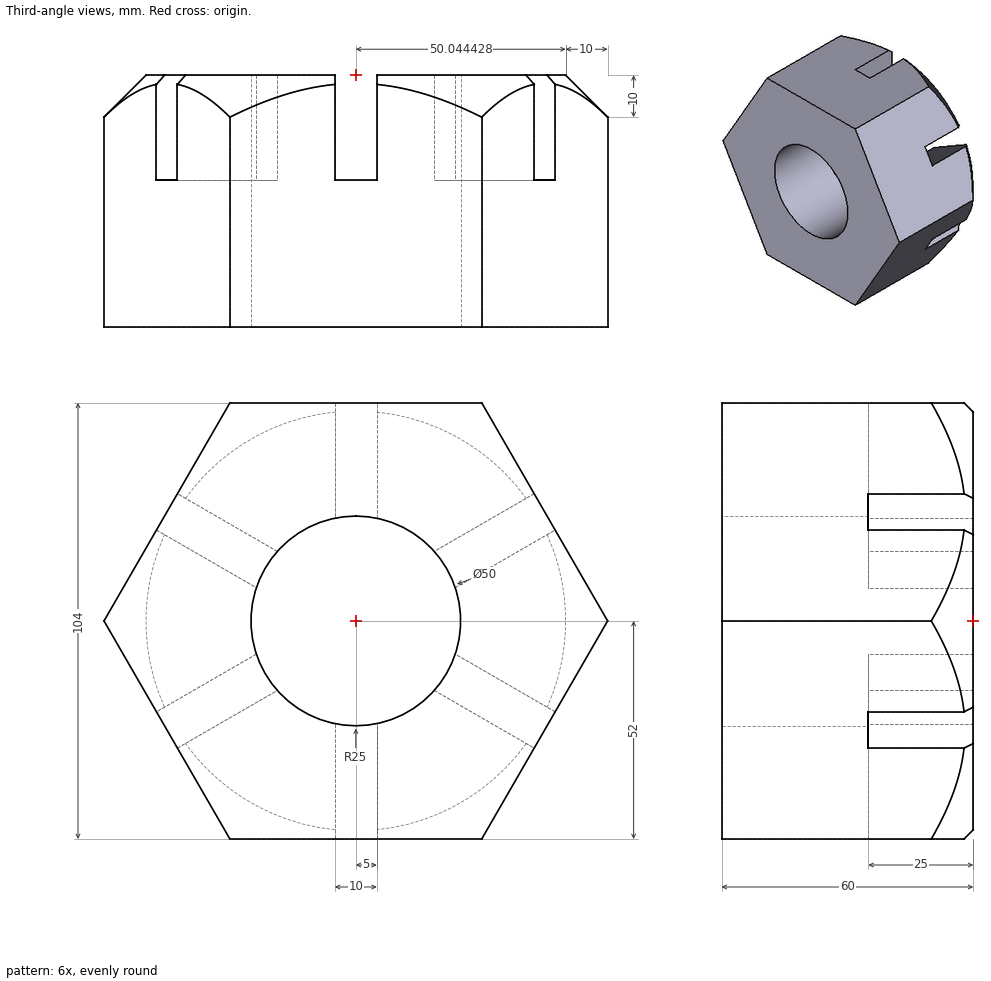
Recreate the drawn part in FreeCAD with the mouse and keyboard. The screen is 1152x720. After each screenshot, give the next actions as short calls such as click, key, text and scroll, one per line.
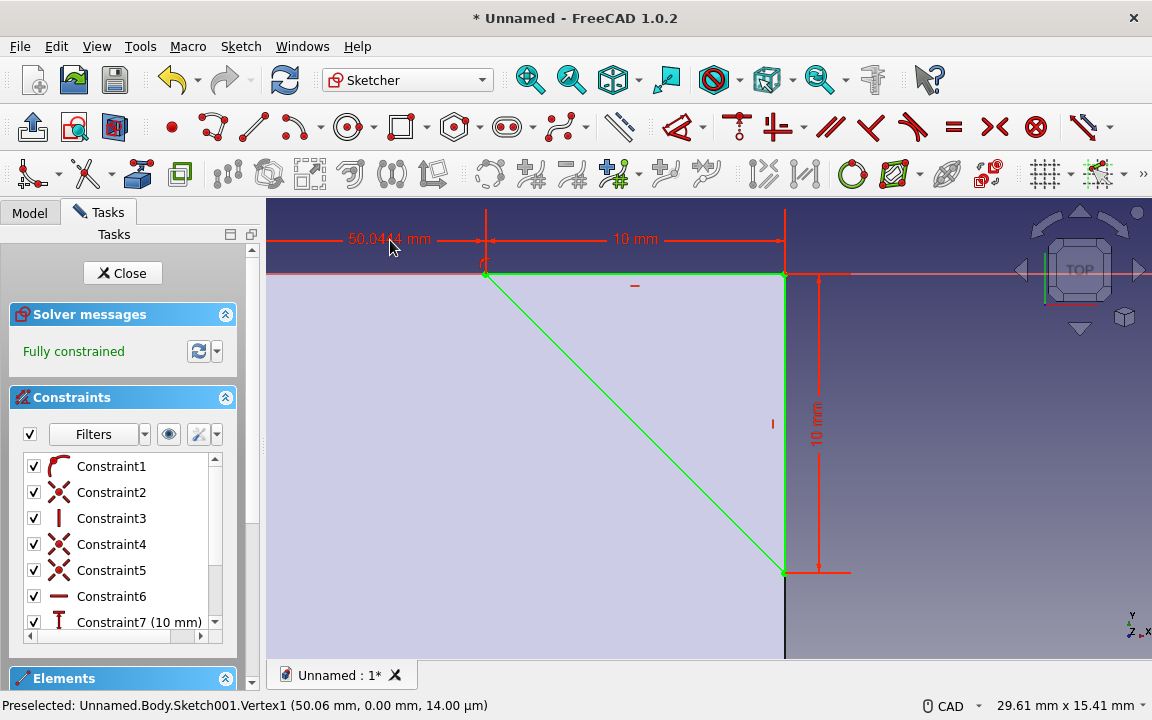
click(123, 273)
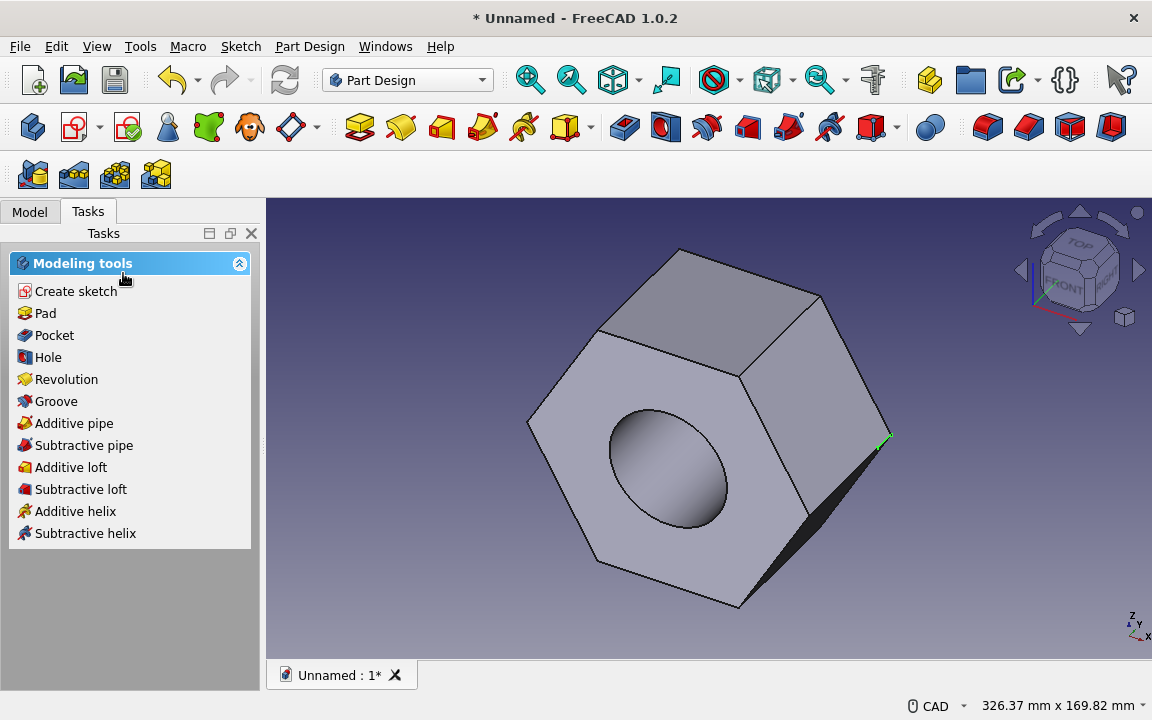
click(707, 128)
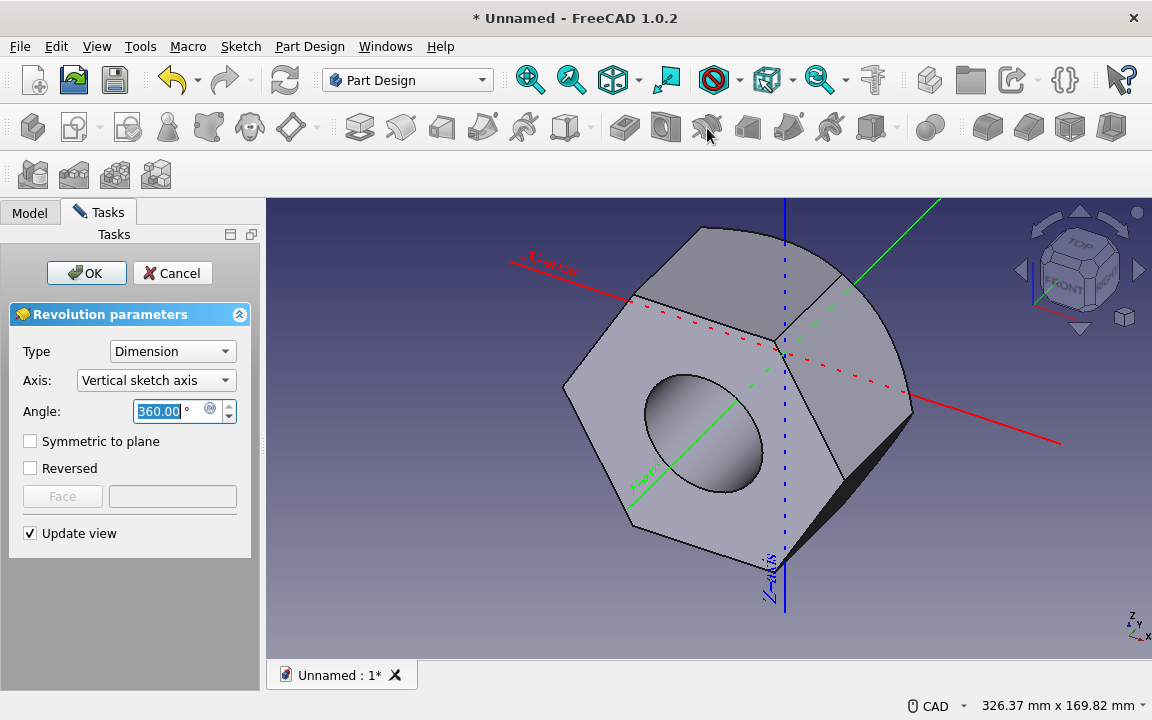
click(87, 273)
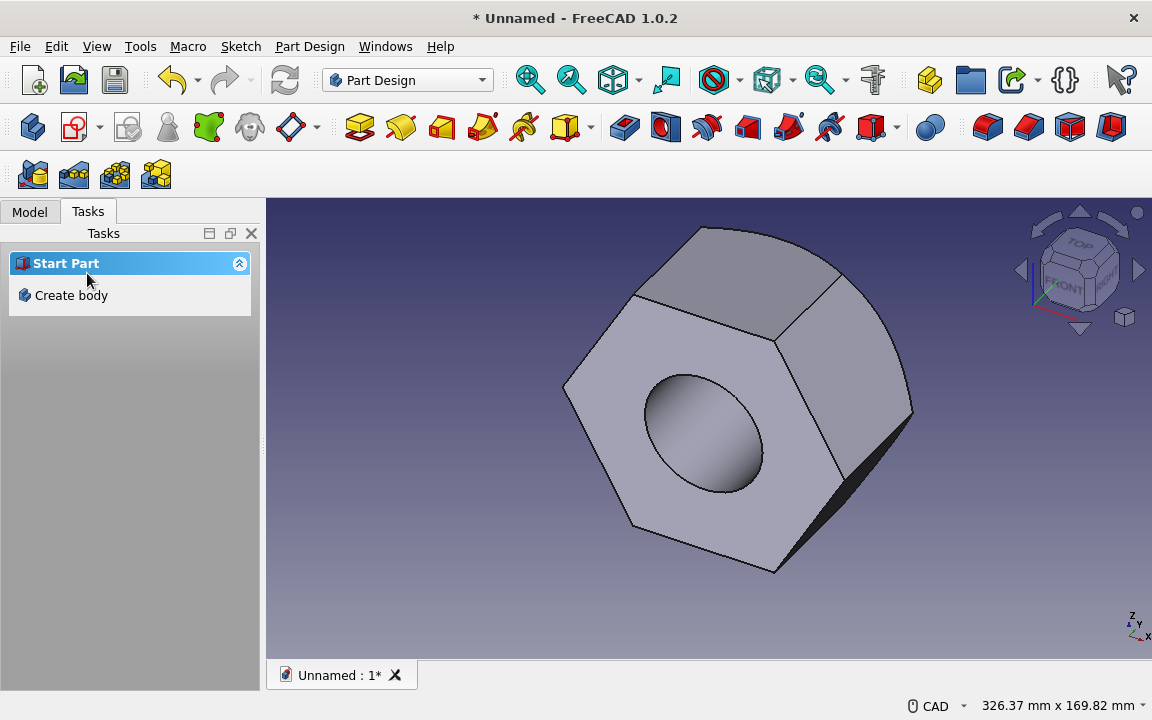
click(531, 80)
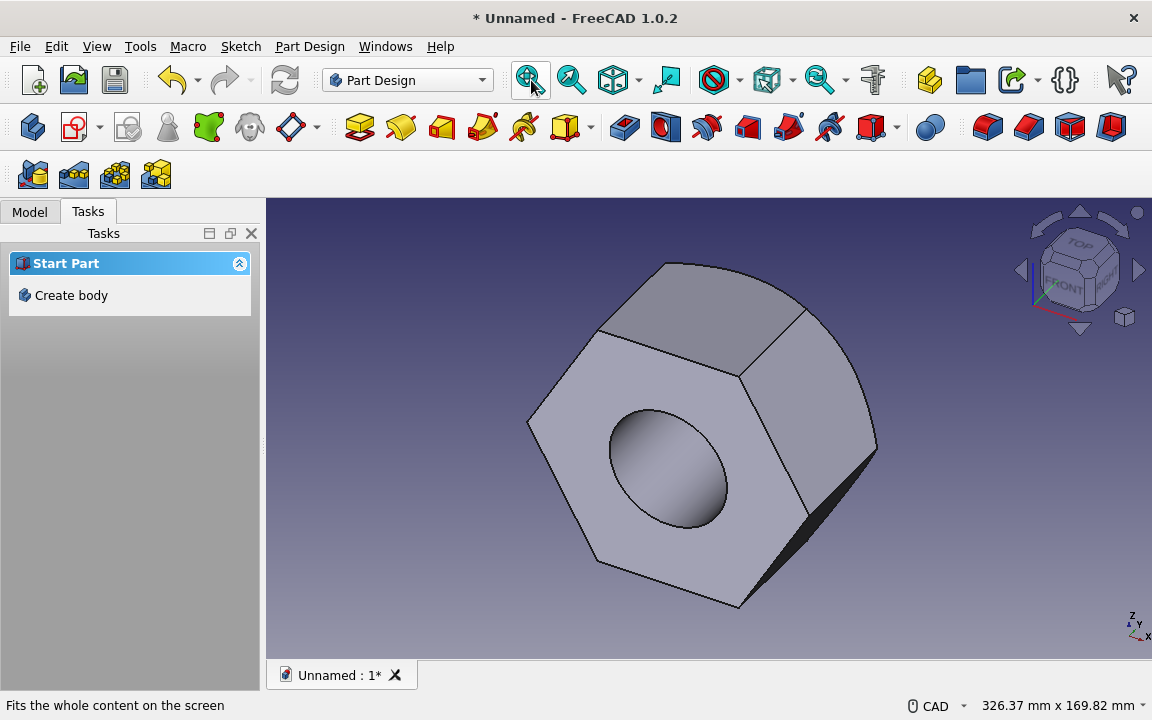
key(4)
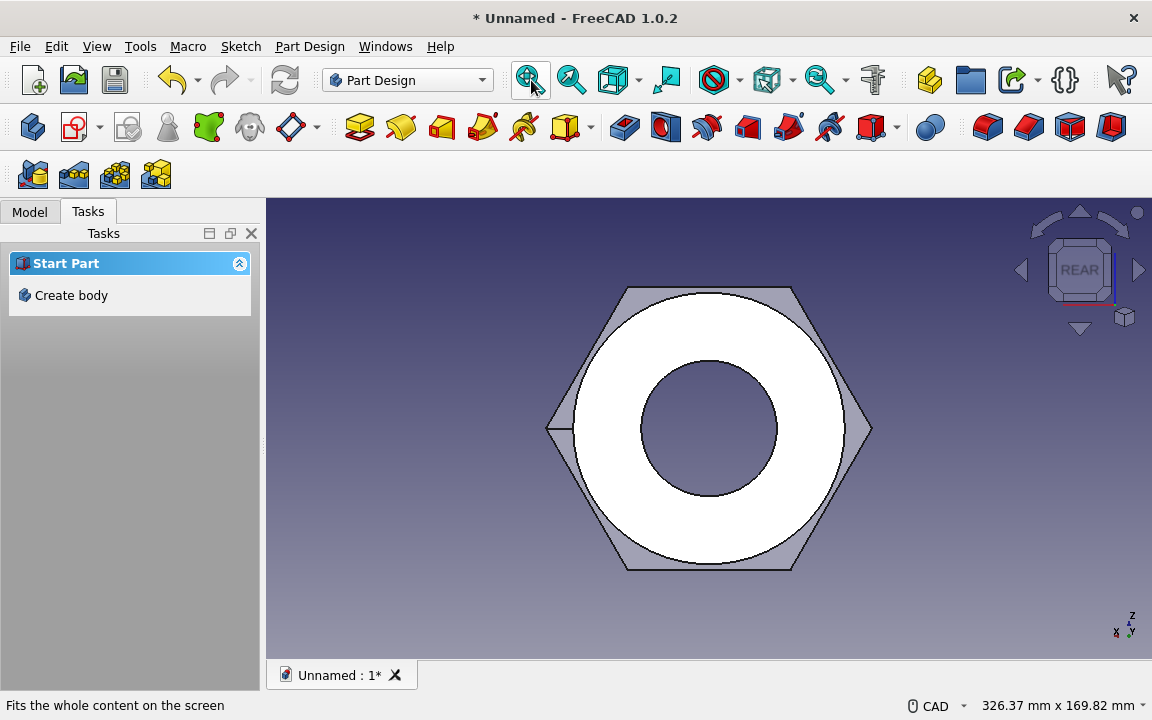
click(787, 350)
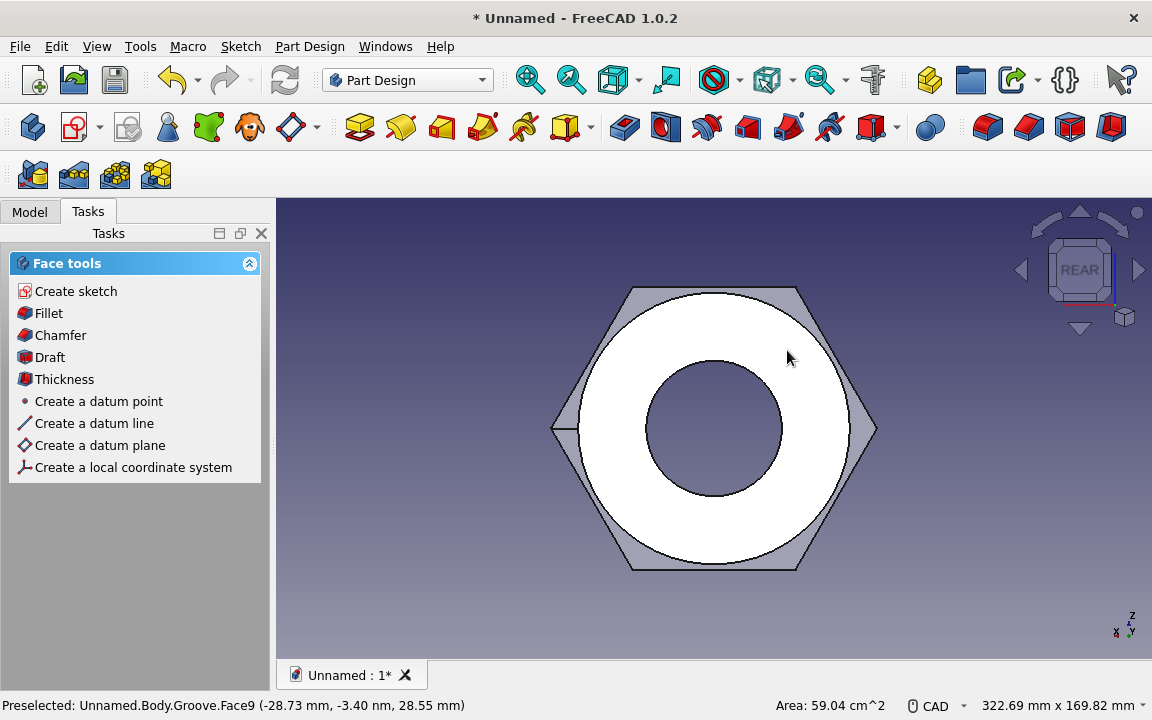
click(74, 128)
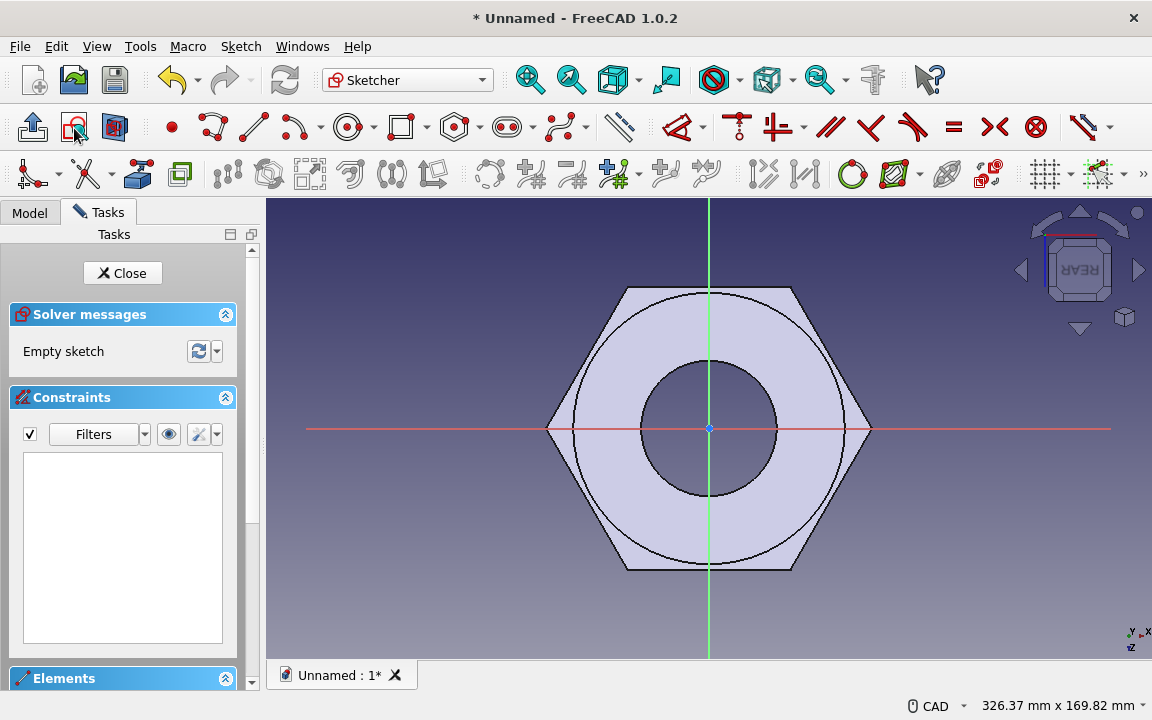
scroll(765, 300, up, 4)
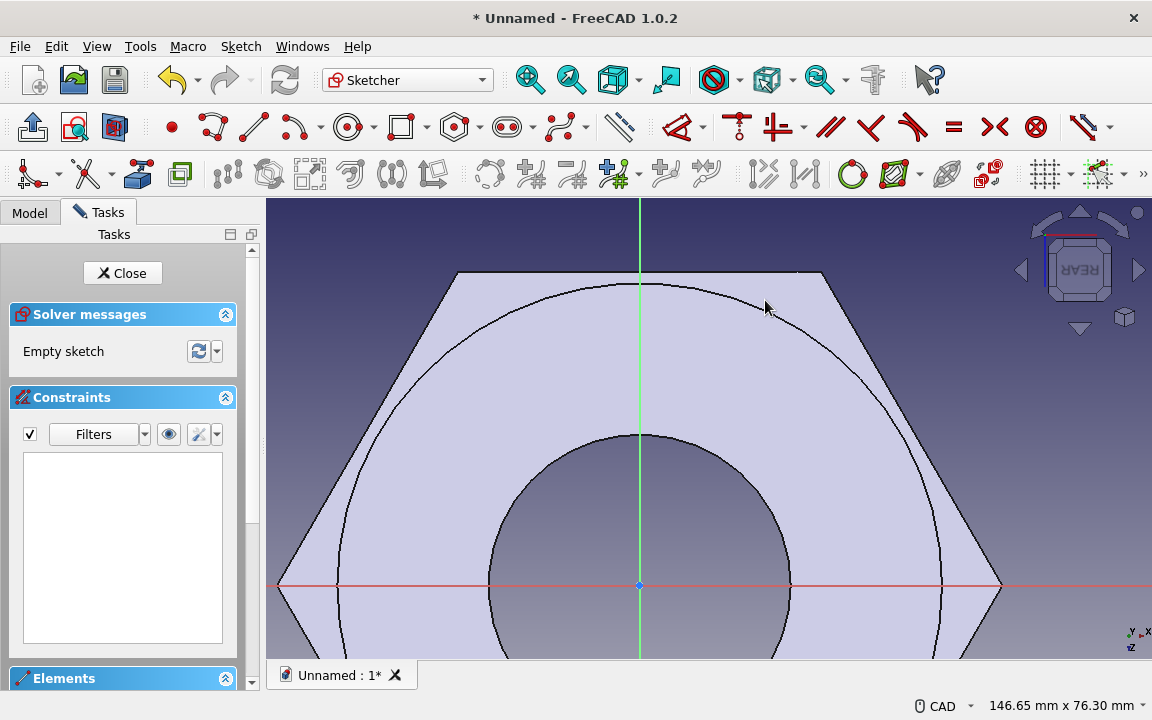
click(213, 128)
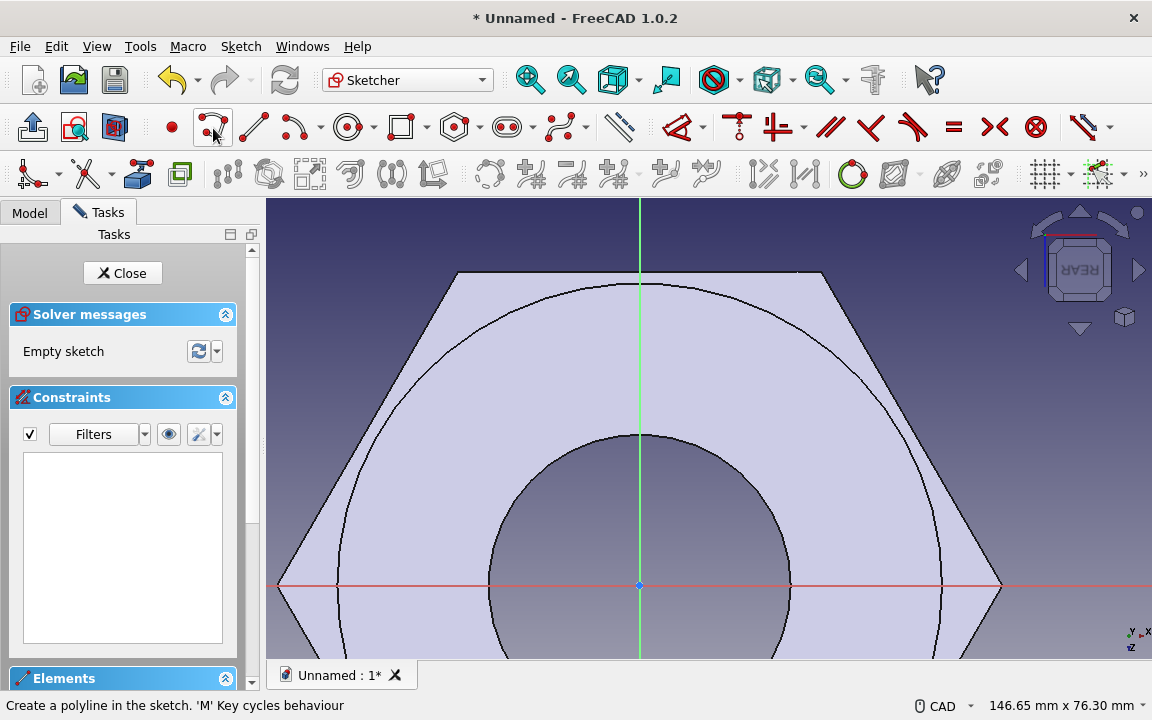
click(670, 438)
click(670, 272)
click(609, 272)
click(609, 438)
right_click(609, 438)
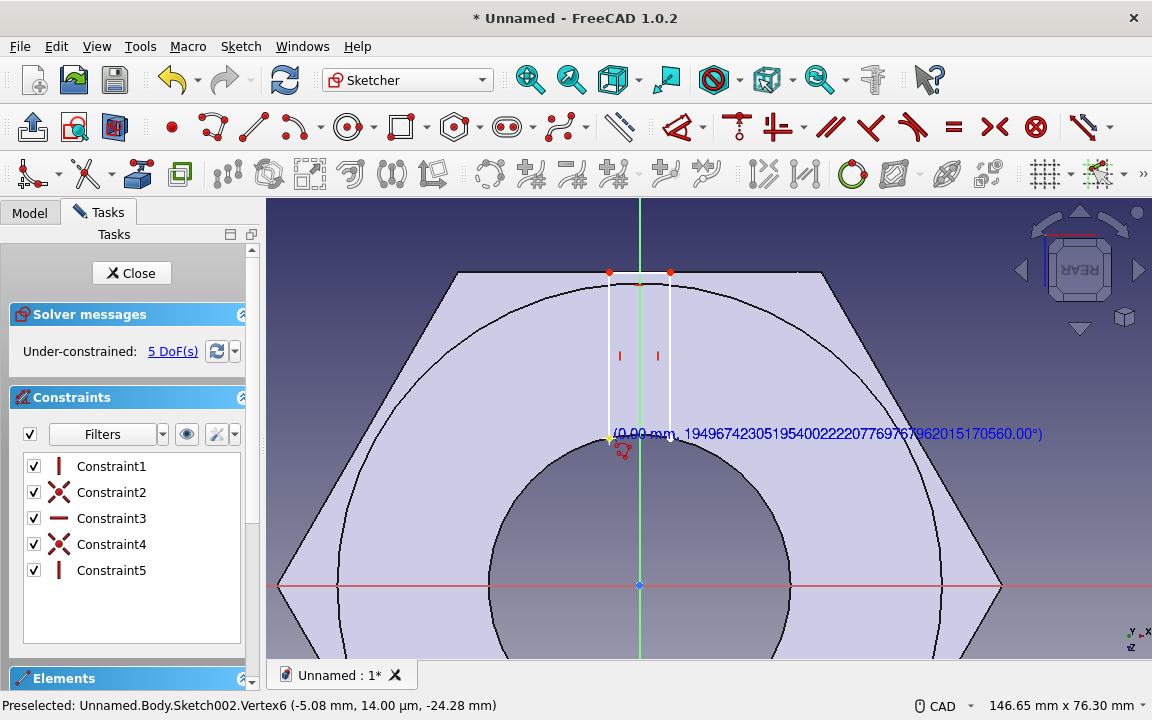
click(320, 128)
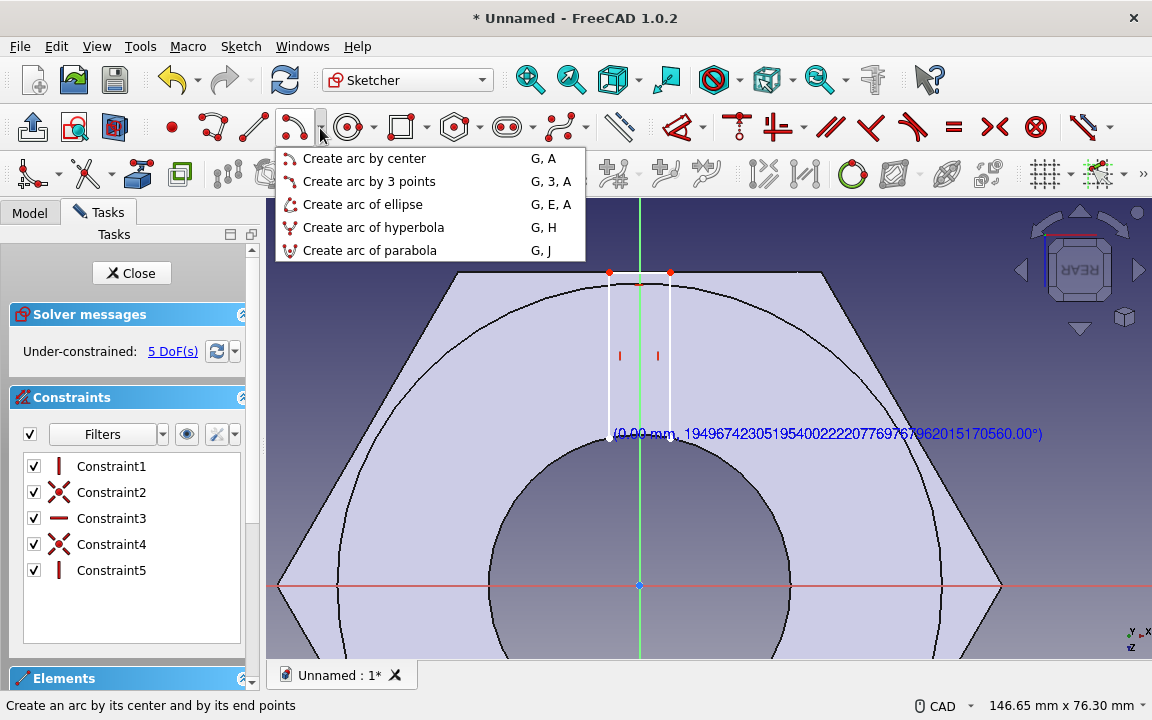
click(430, 182)